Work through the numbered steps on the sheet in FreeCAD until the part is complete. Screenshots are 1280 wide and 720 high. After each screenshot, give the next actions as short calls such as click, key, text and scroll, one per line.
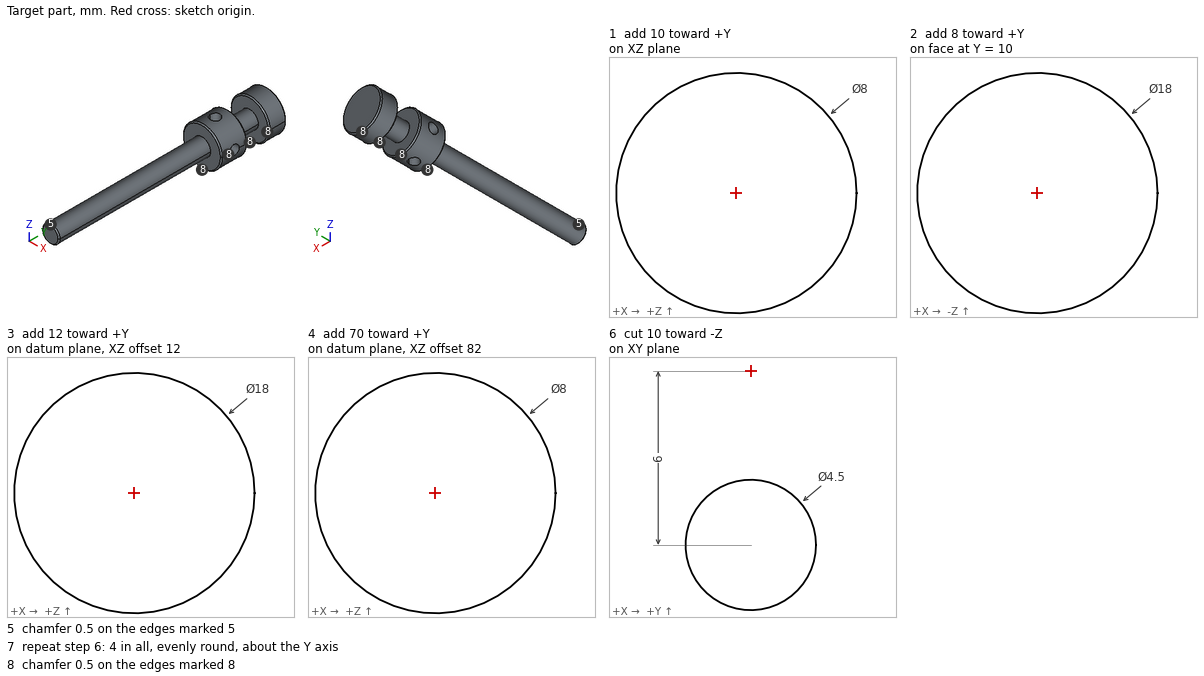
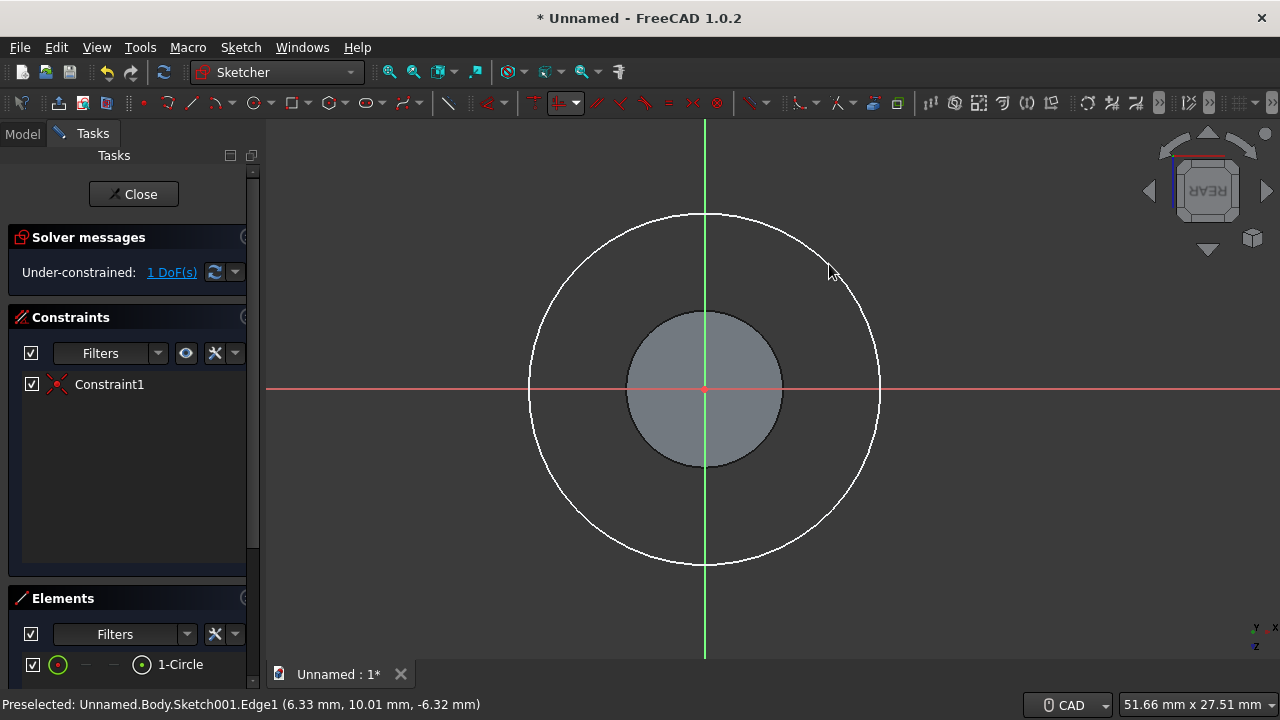
click(488, 104)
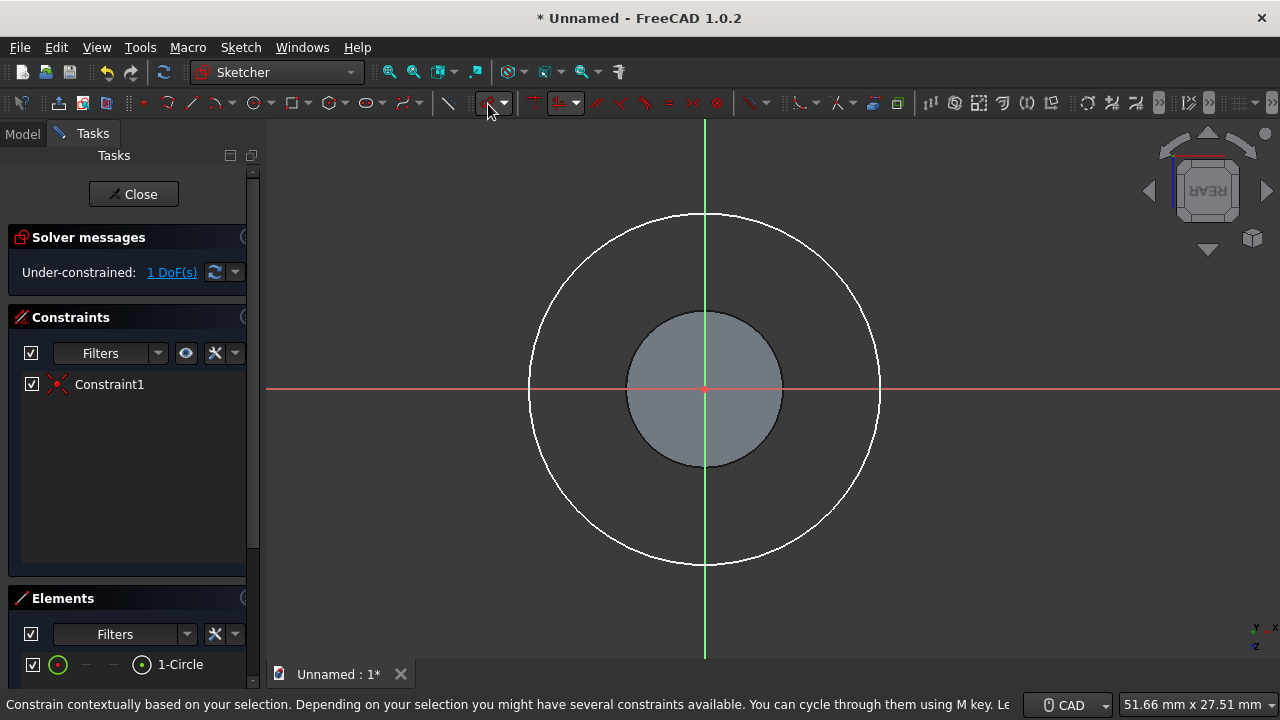
click(829, 265)
click(852, 242)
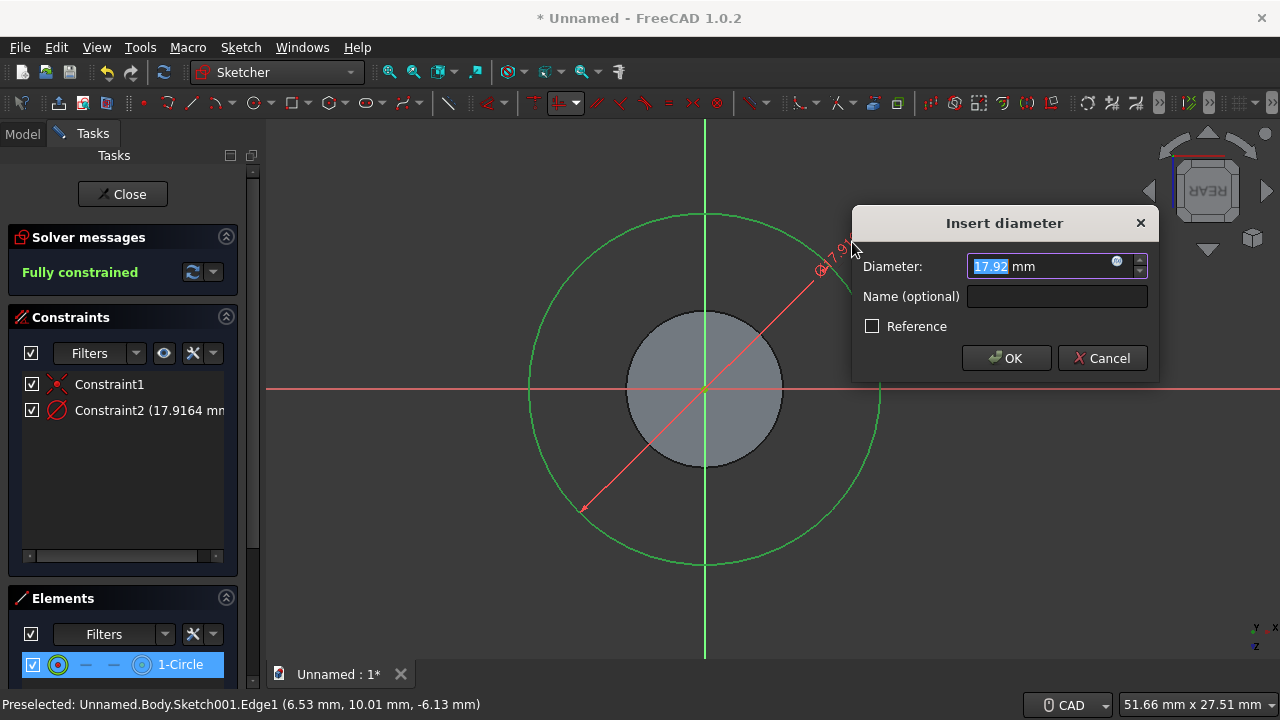
text(18)
key(Return)
key(Escape)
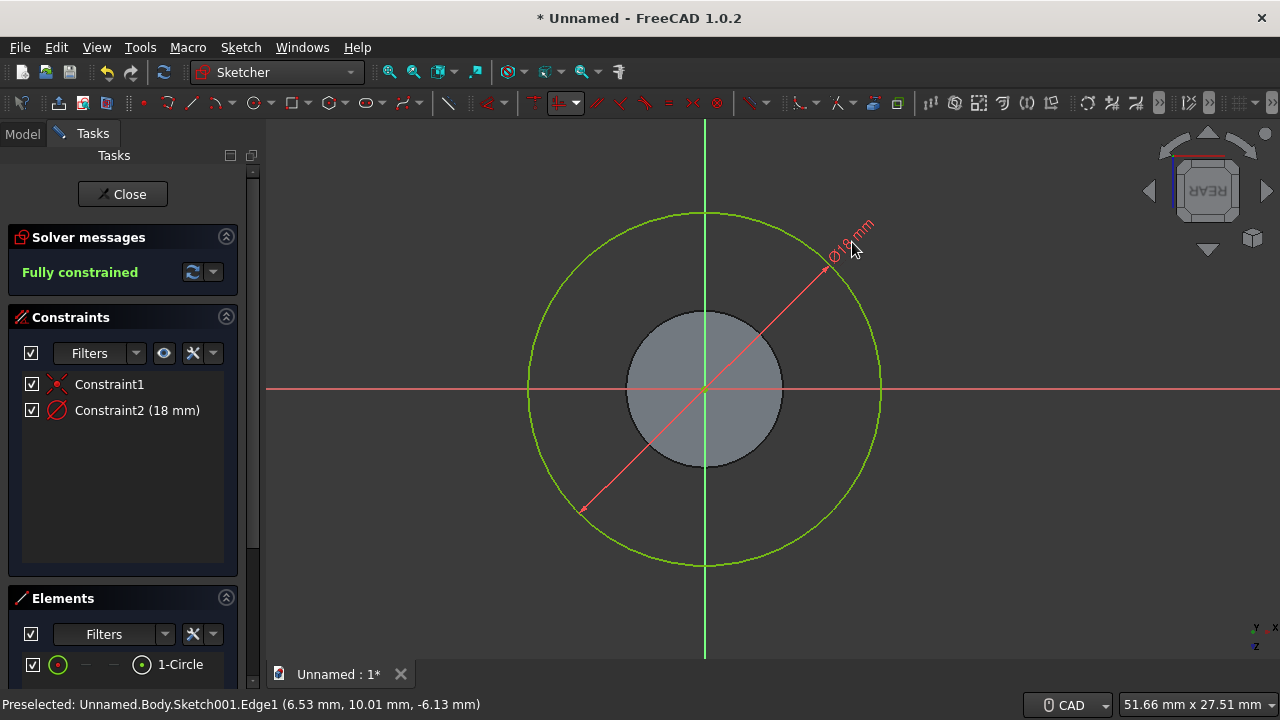
click(123, 194)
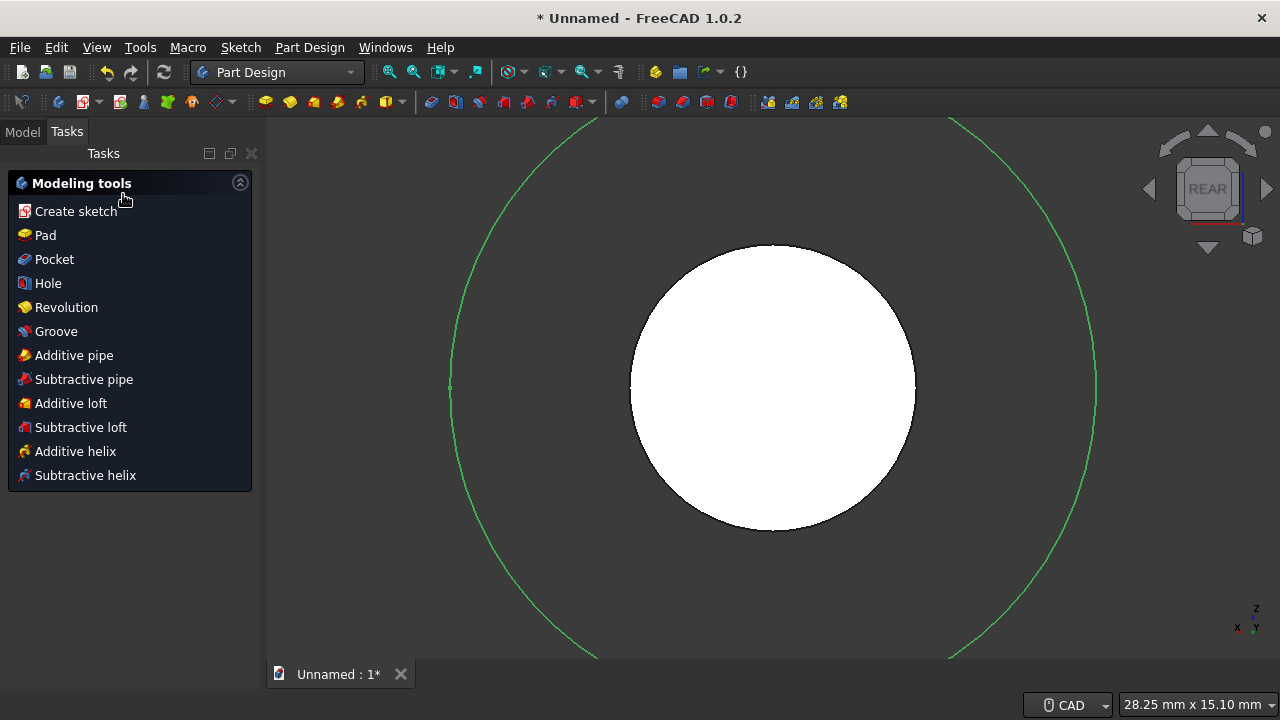
click(266, 102)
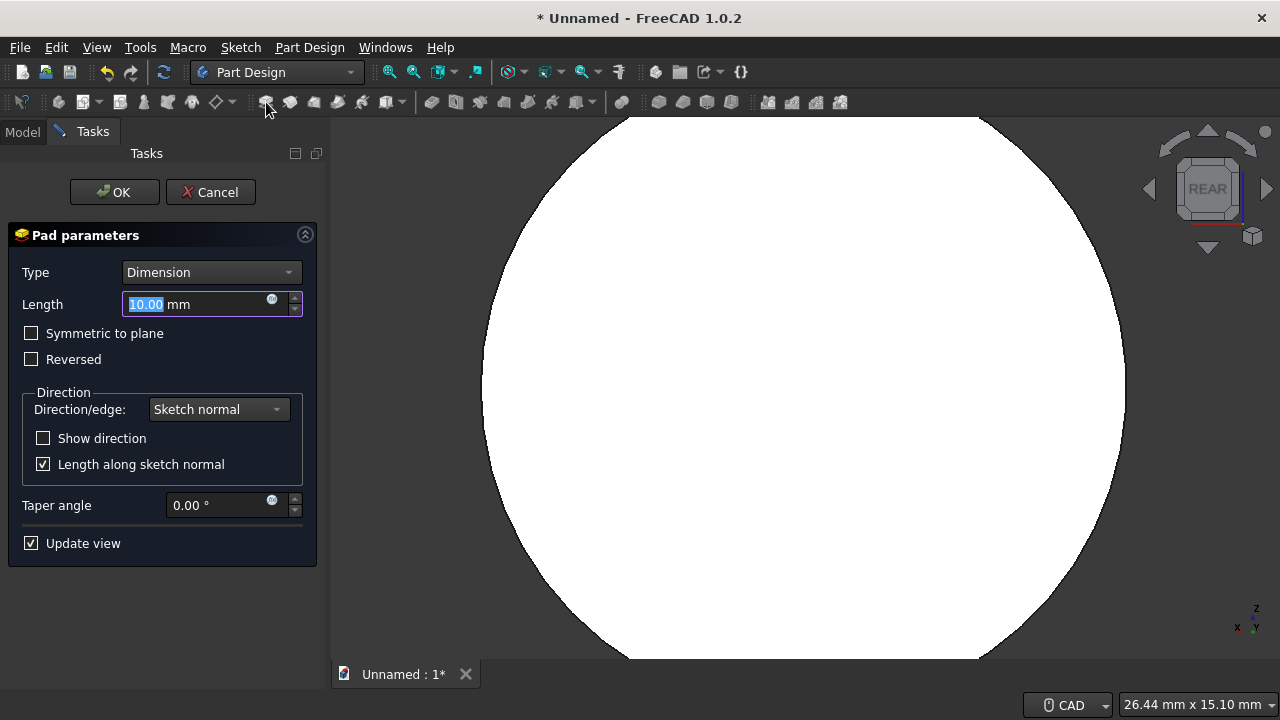
text(8)
key(Tab)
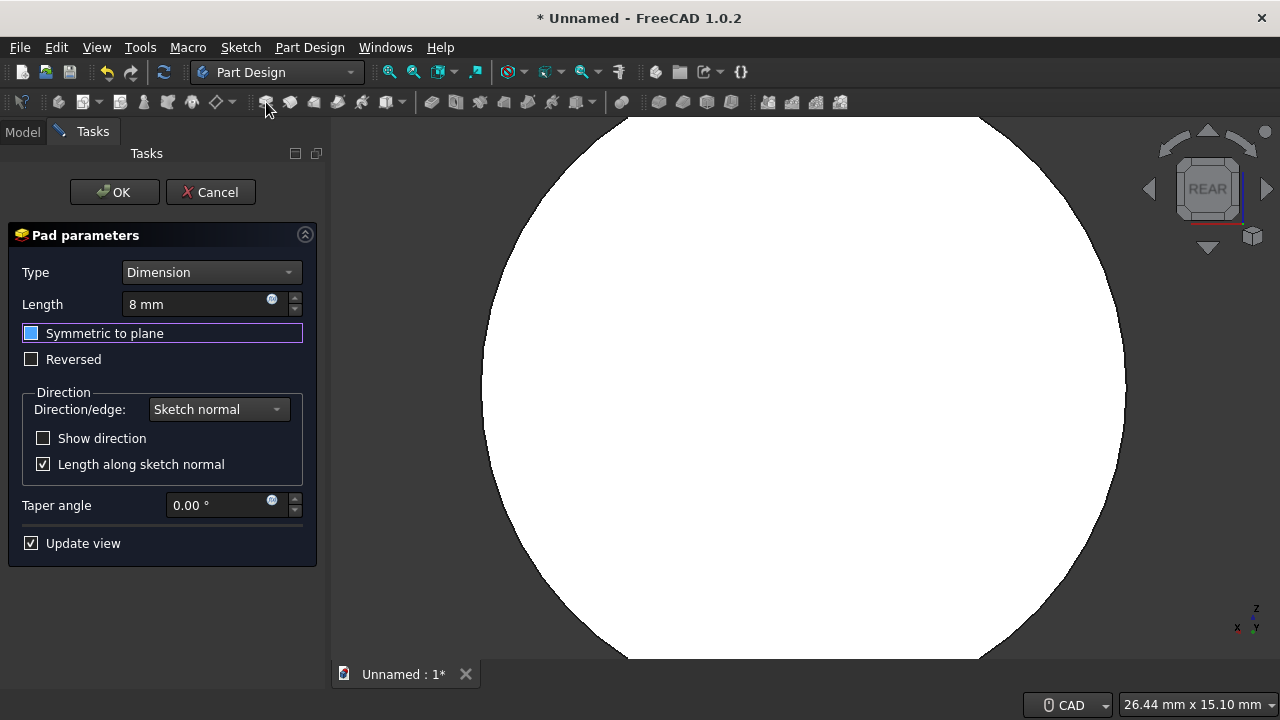
click(115, 192)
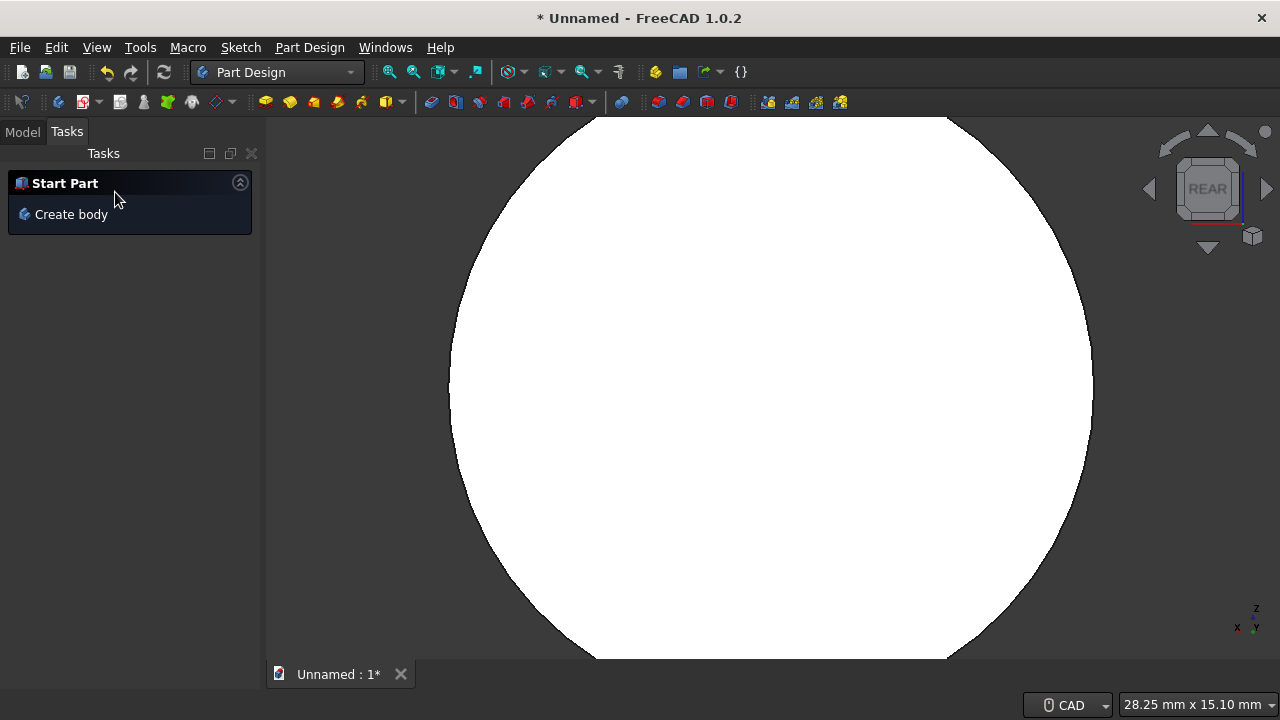
click(390, 72)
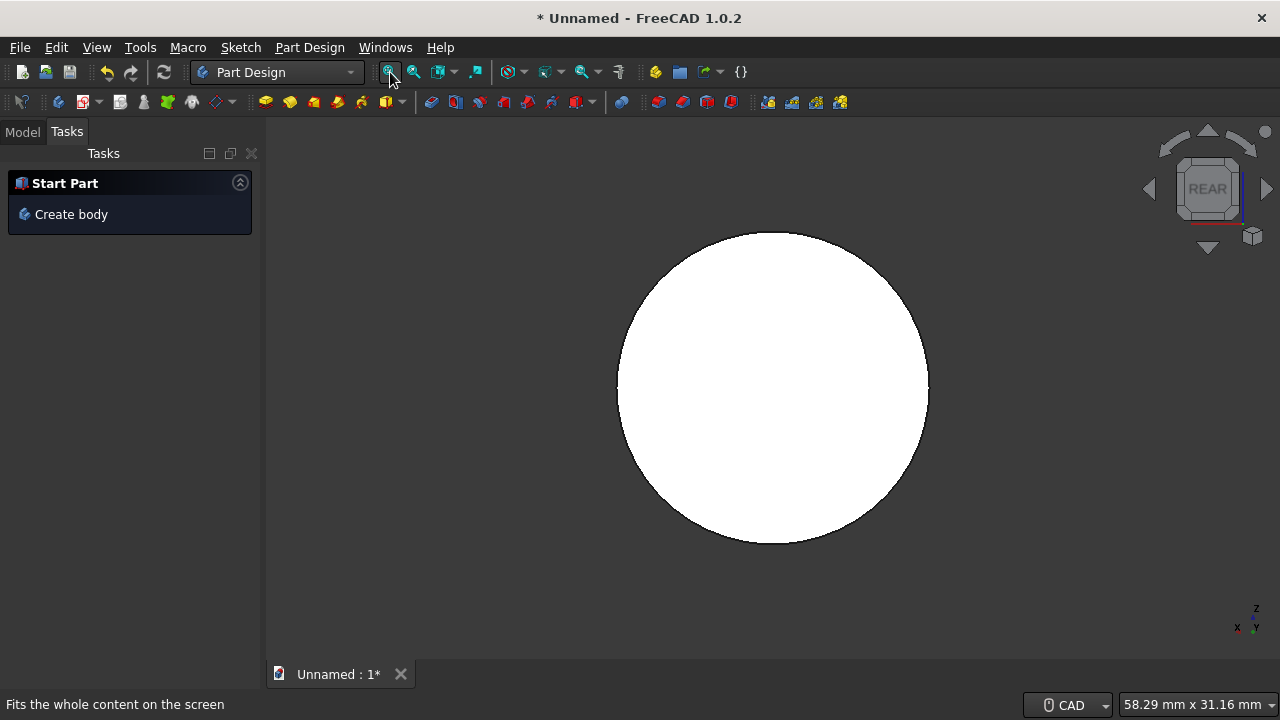
click(23, 131)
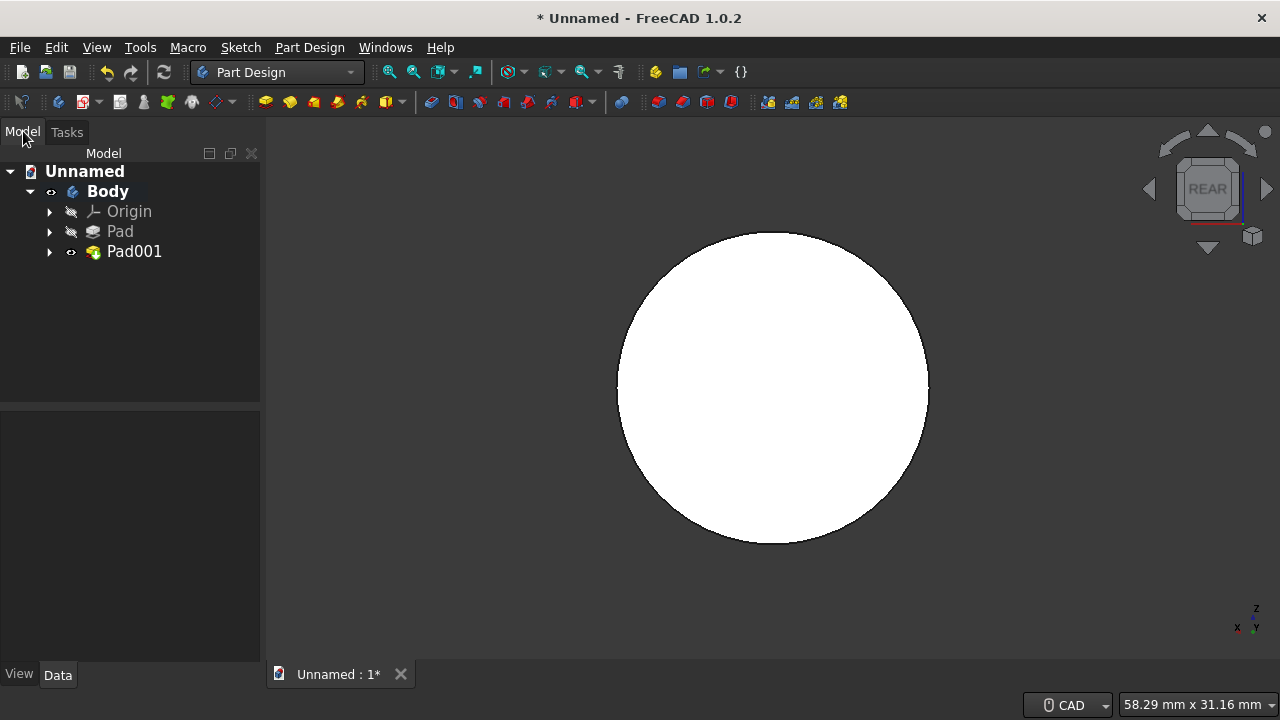
click(50, 212)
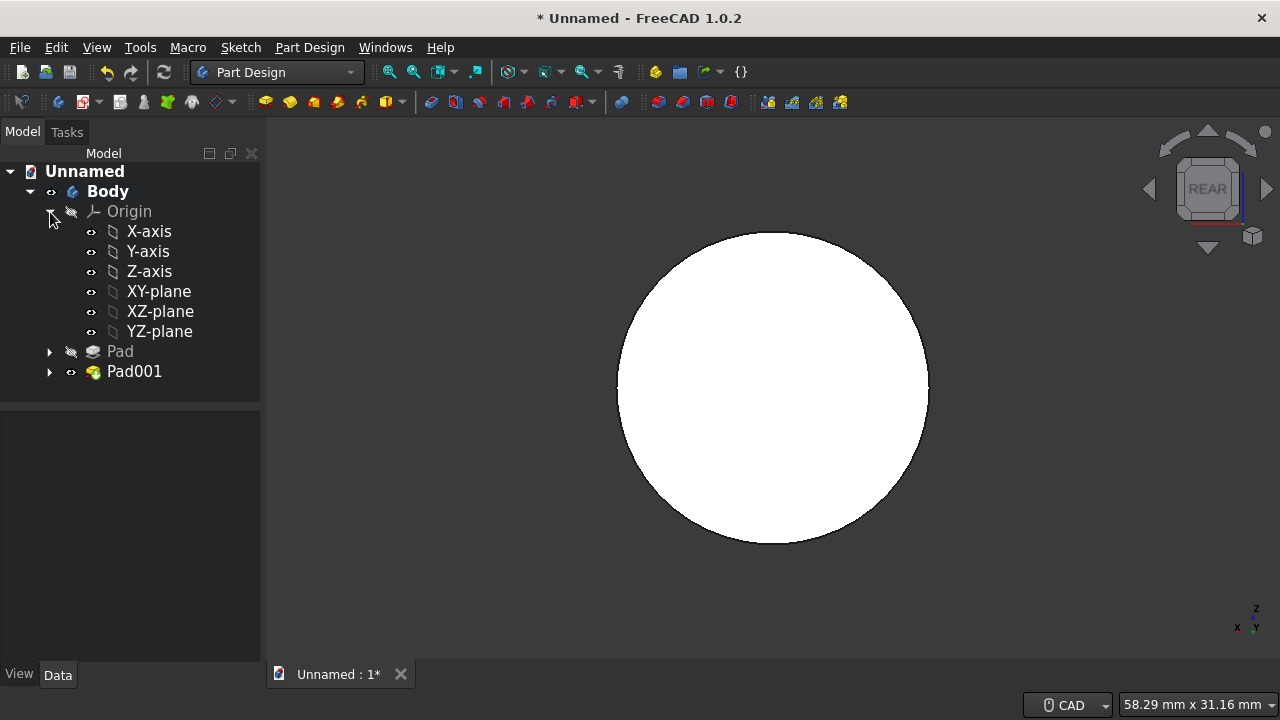
click(136, 312)